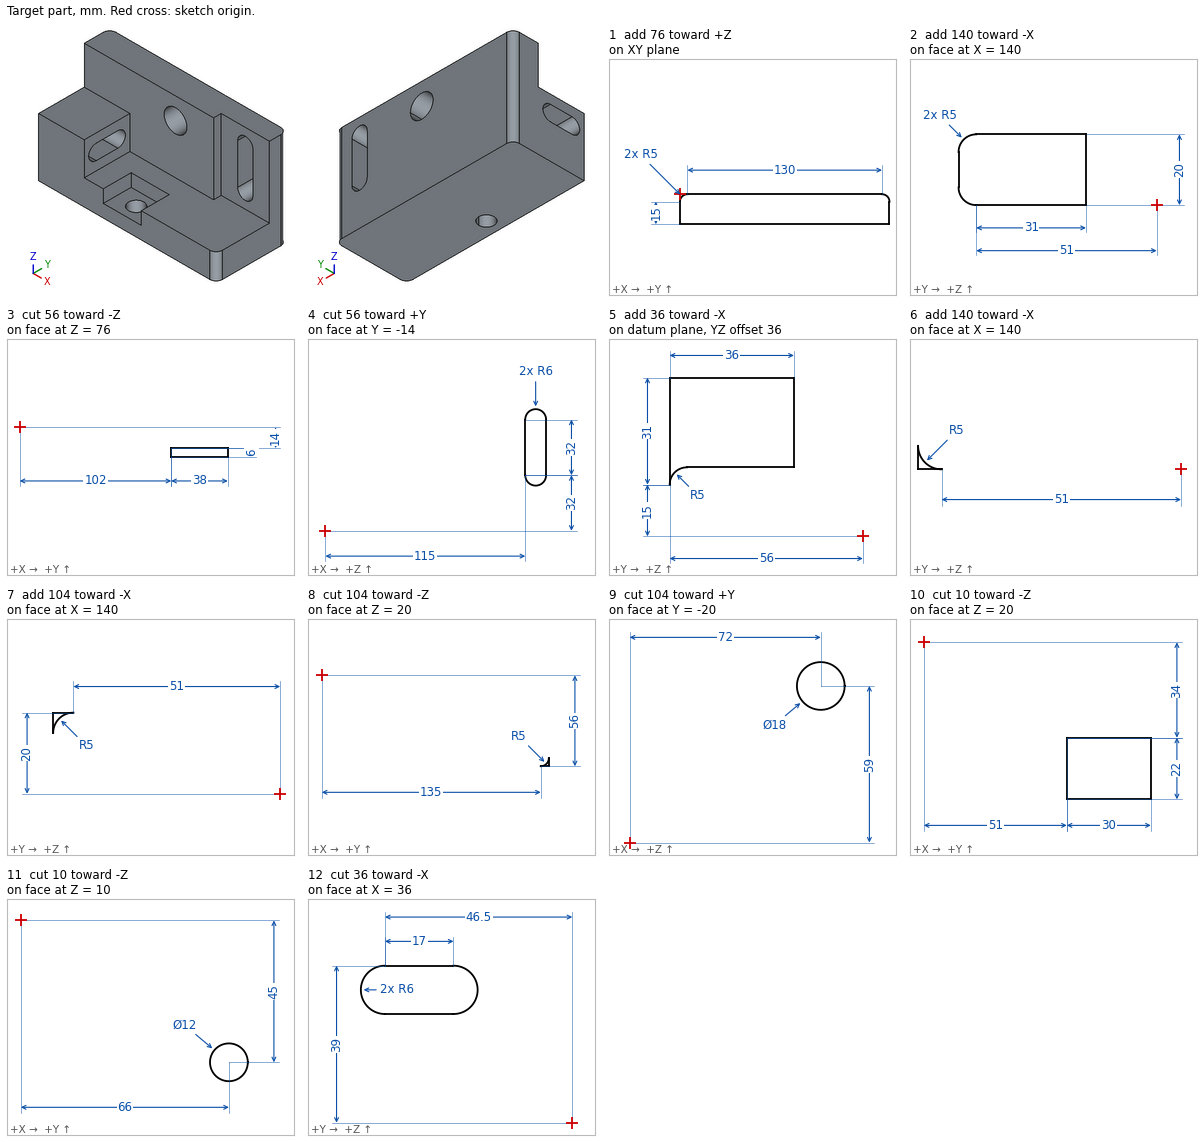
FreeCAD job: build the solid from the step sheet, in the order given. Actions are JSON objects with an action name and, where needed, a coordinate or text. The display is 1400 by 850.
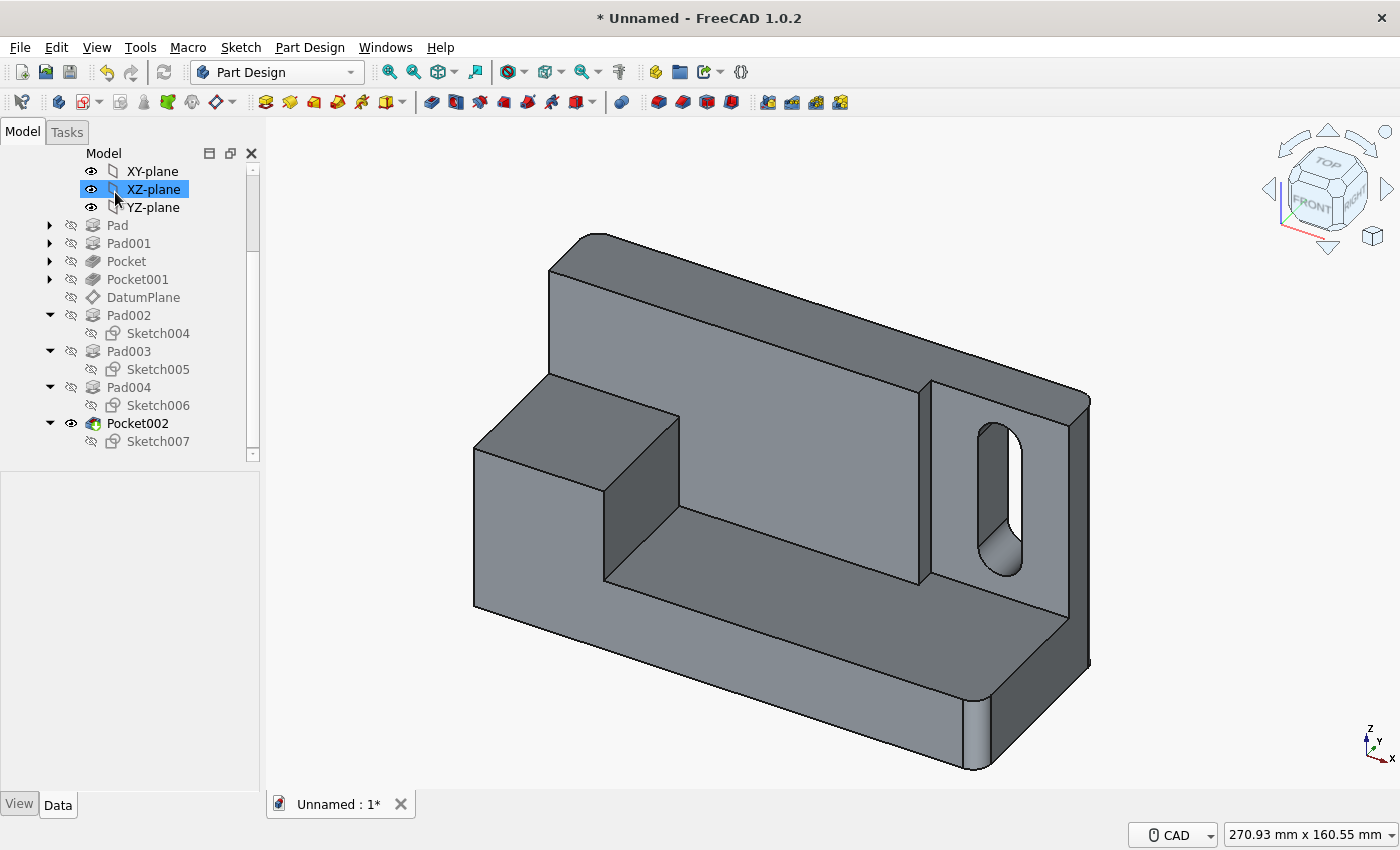
{"action": "left_click", "coordinate": [787, 444]}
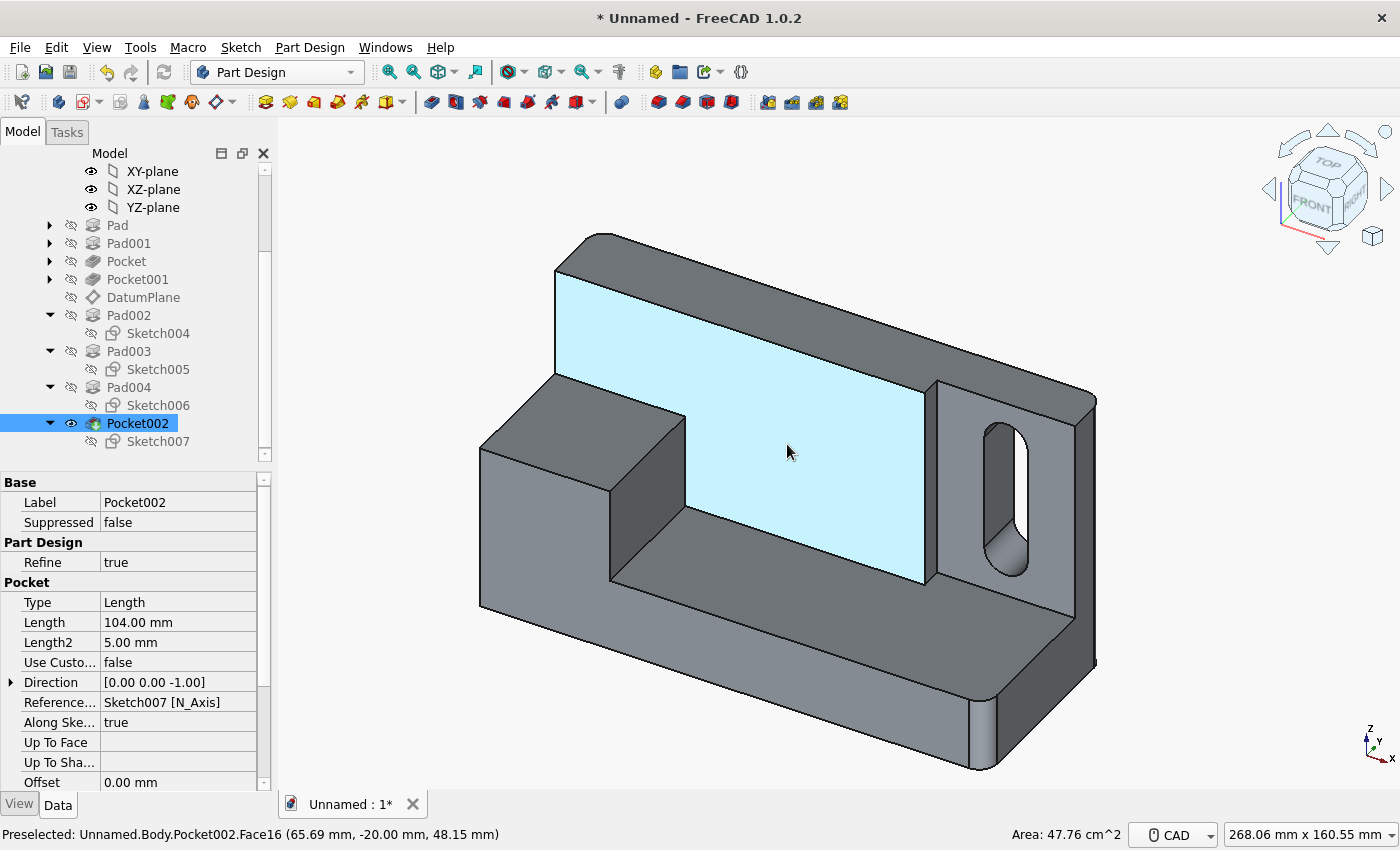
{"action": "left_click", "coordinate": [84, 102]}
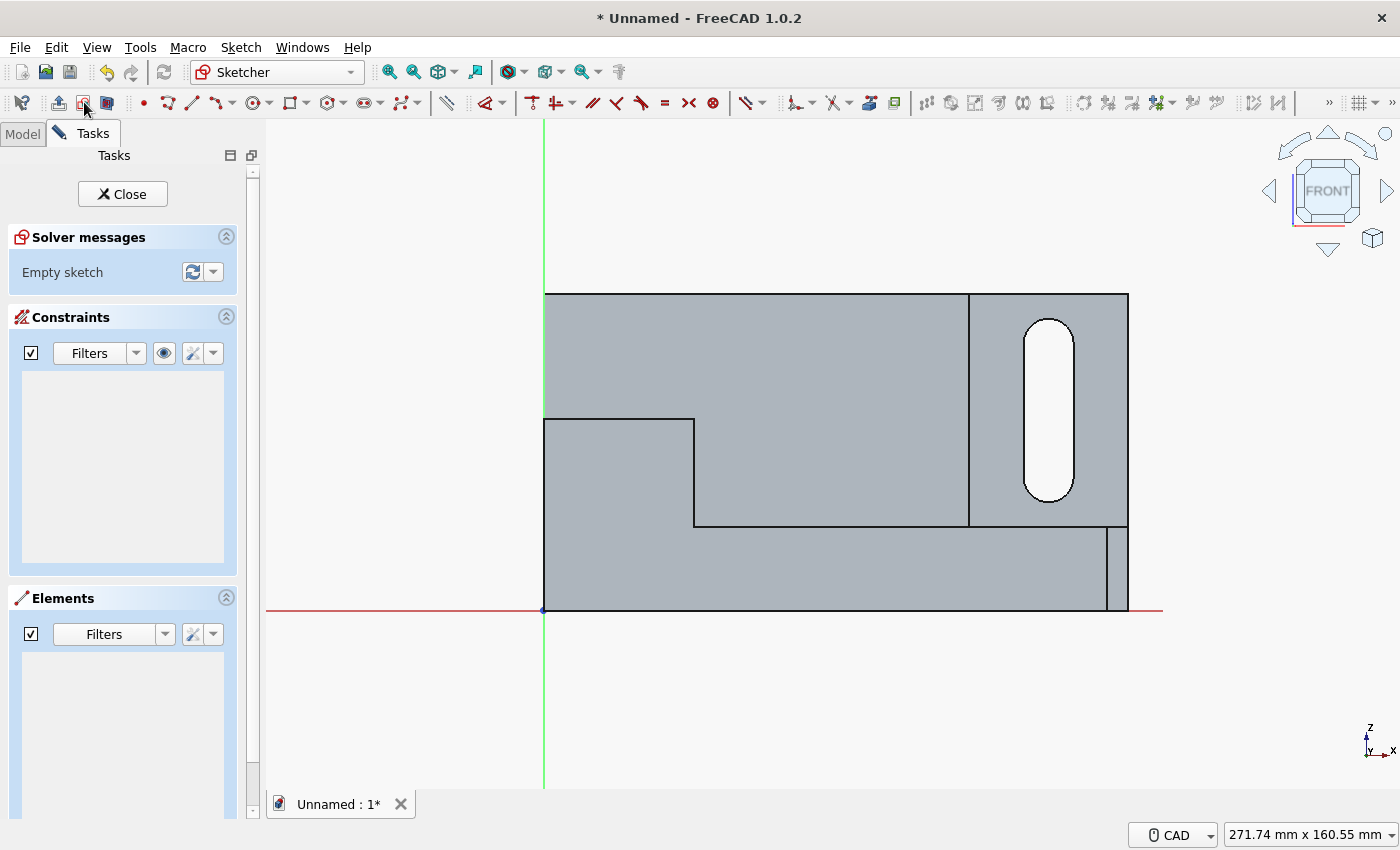
{"action": "scroll", "coordinate": [860, 347], "scroll_direction": "up", "scroll_amount": 9}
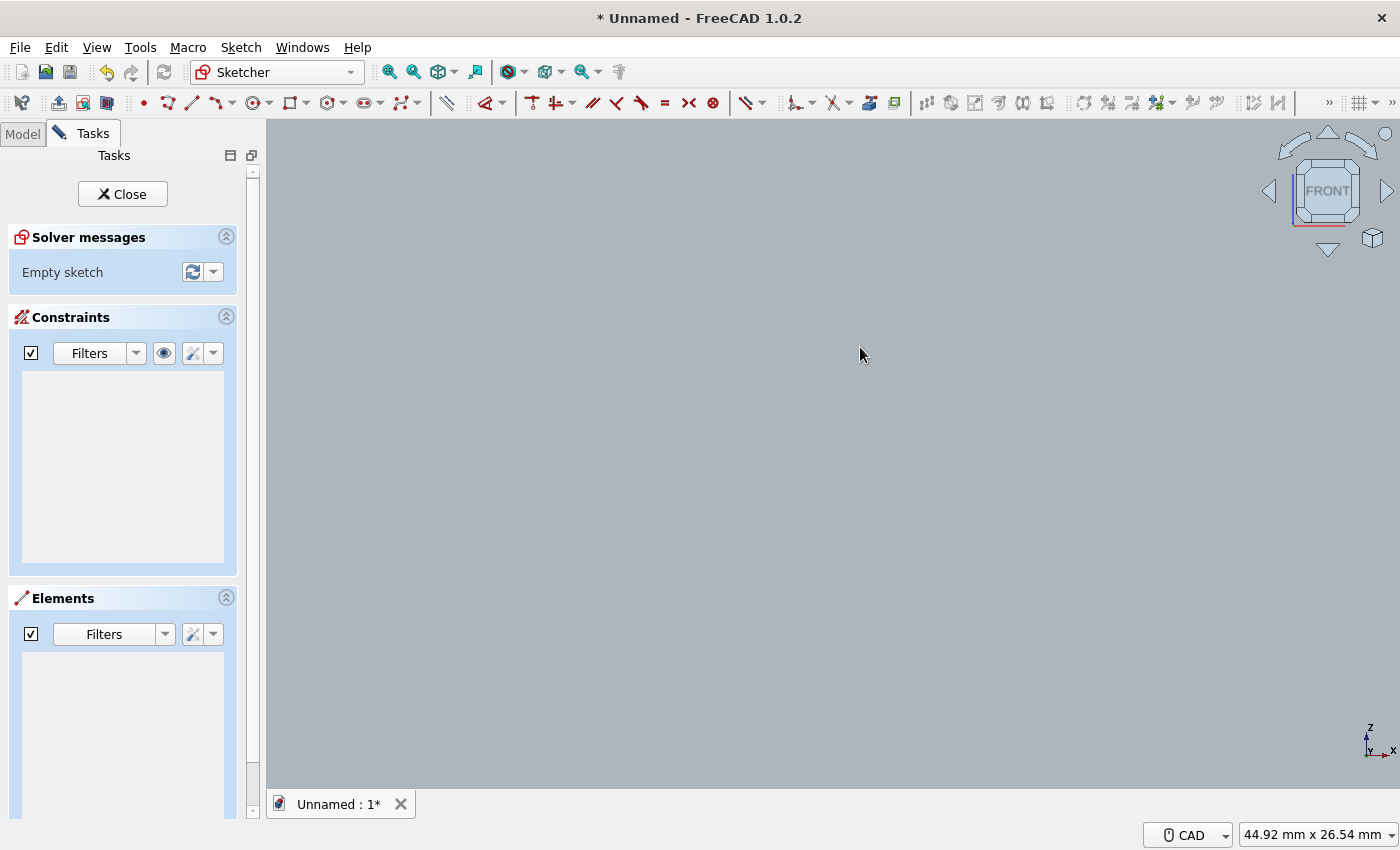
{"action": "left_click", "coordinate": [254, 104]}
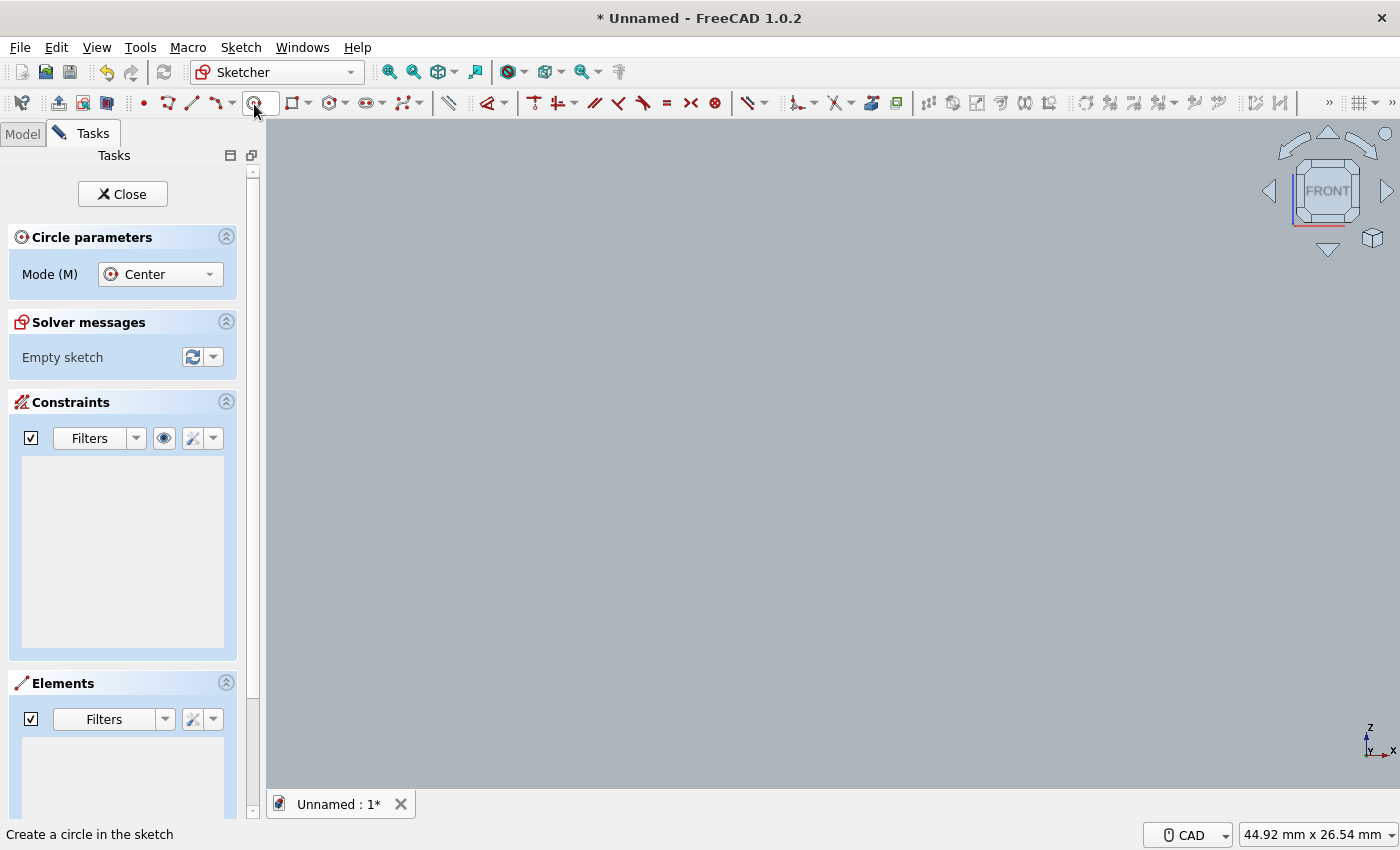
{"action": "left_click", "coordinate": [762, 451]}
{"action": "left_click", "coordinate": [922, 291]}
{"action": "key", "text": "Escape"}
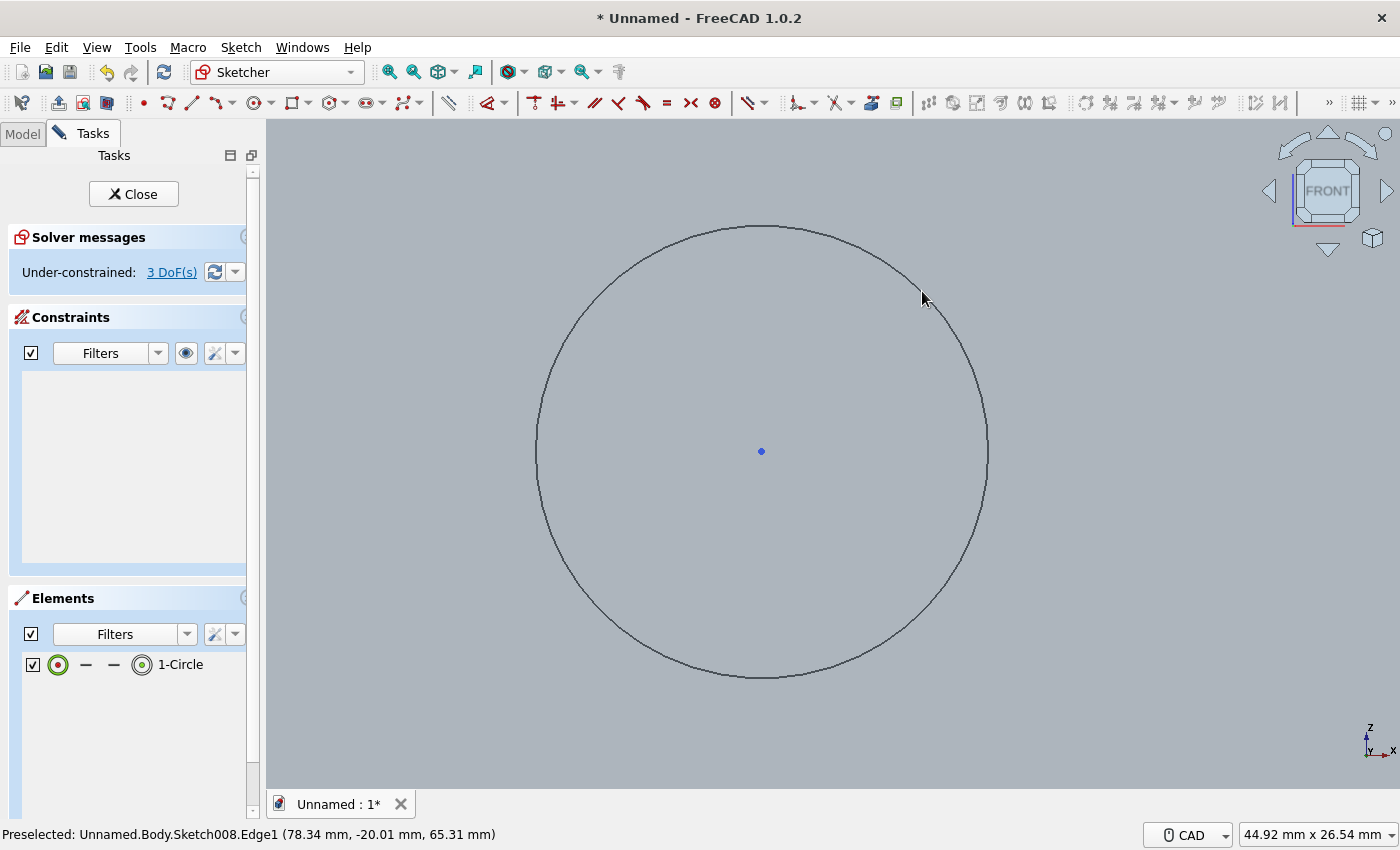
{"action": "left_click", "coordinate": [488, 104]}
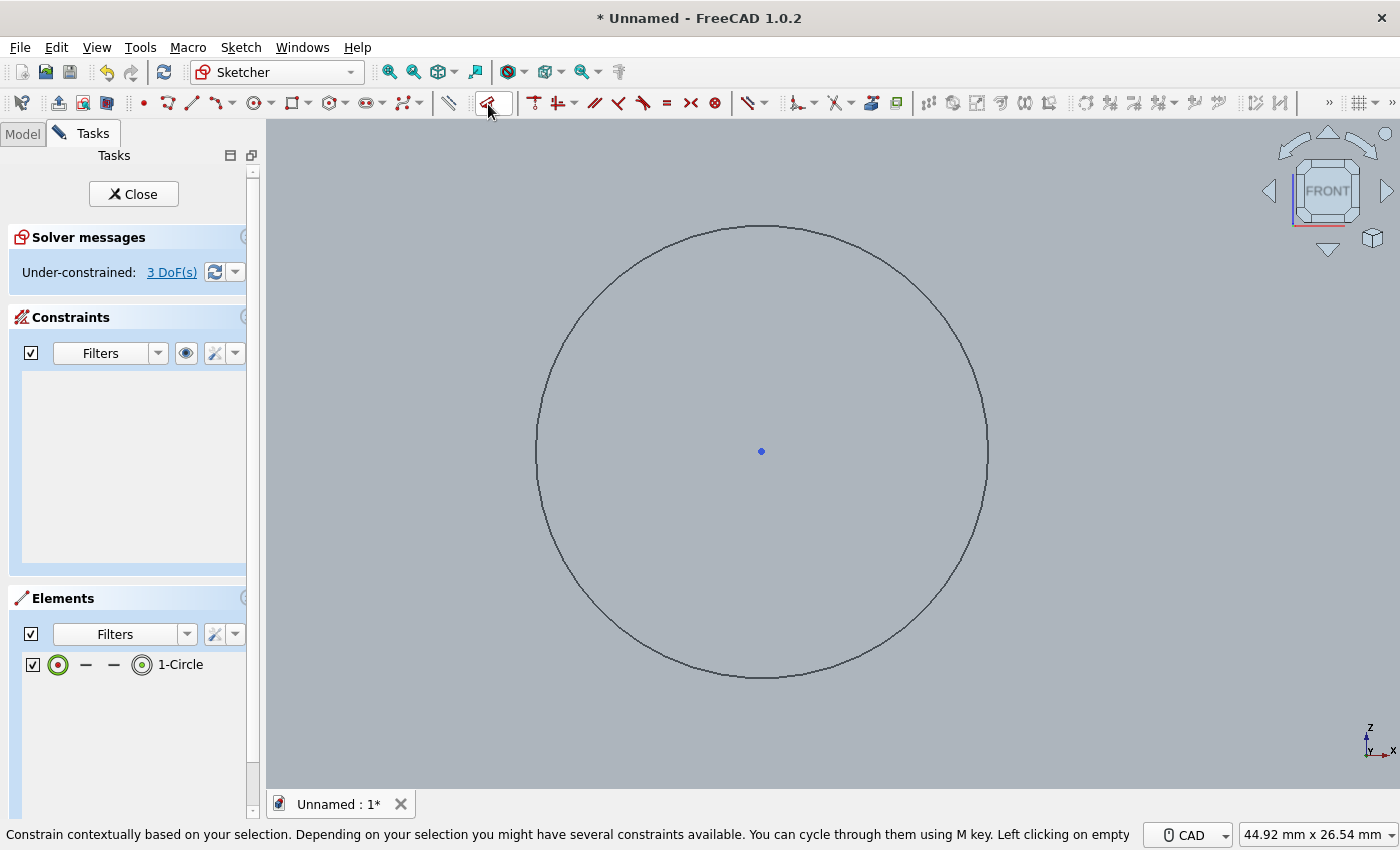
{"action": "left_click", "coordinate": [922, 292]}
{"action": "left_click", "coordinate": [945, 269]}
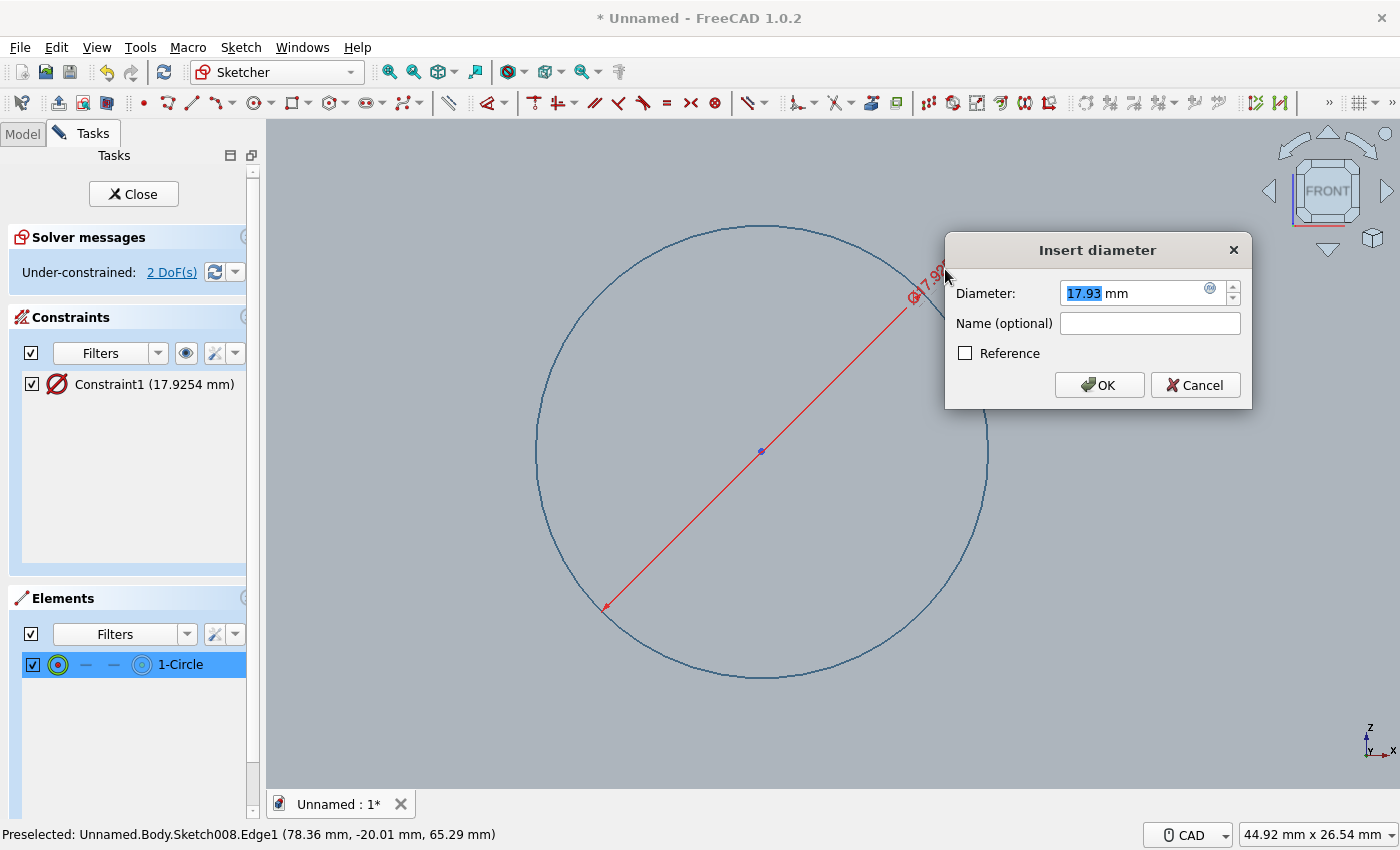
{"action": "type", "text": "18"}
{"action": "key", "text": "Return"}